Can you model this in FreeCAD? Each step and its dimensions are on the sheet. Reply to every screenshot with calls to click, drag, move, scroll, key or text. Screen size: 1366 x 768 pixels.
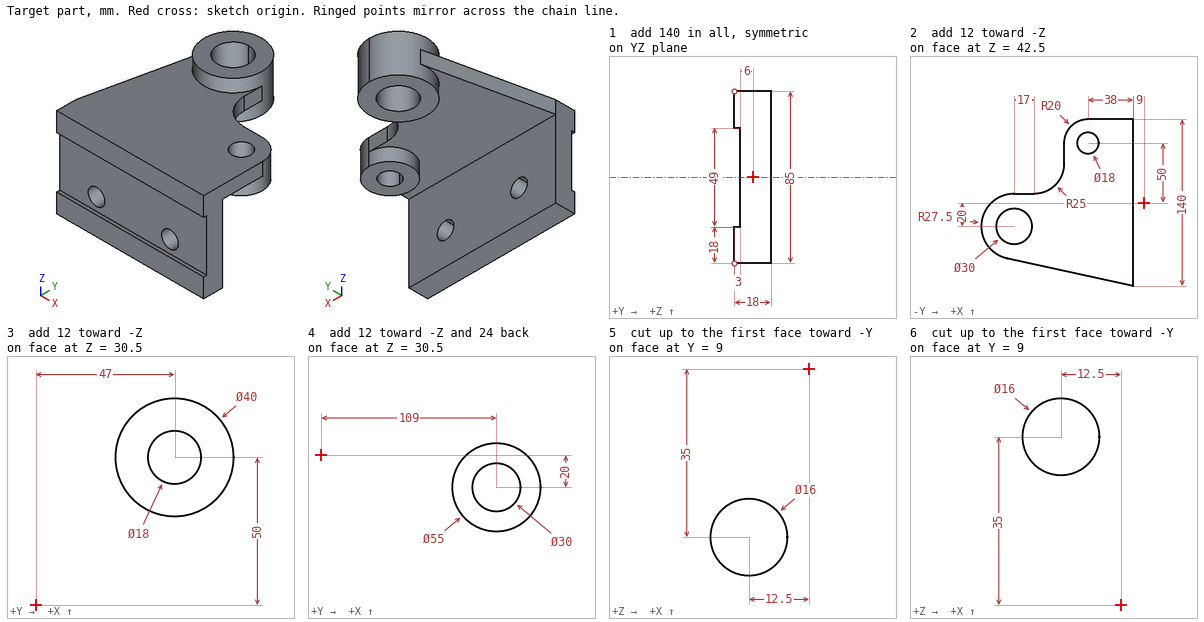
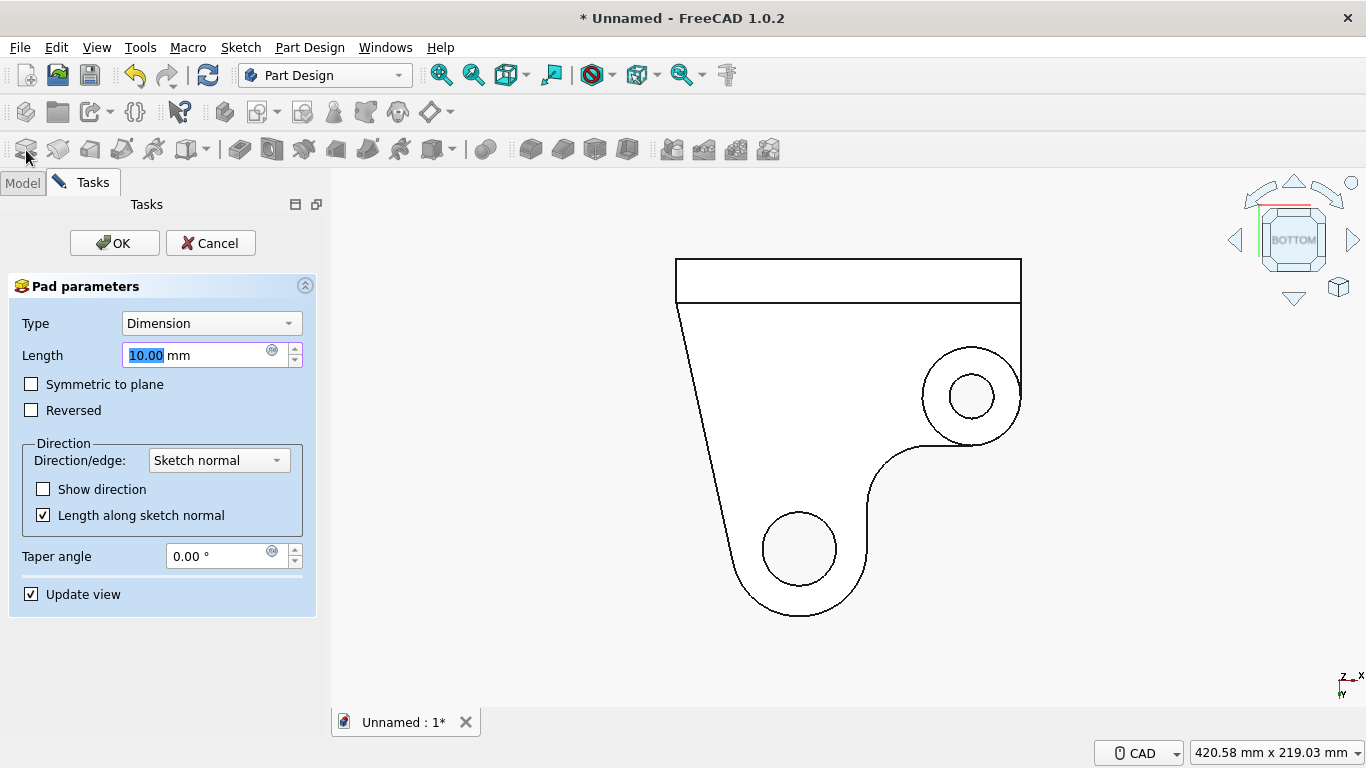
text(12)
key(Tab)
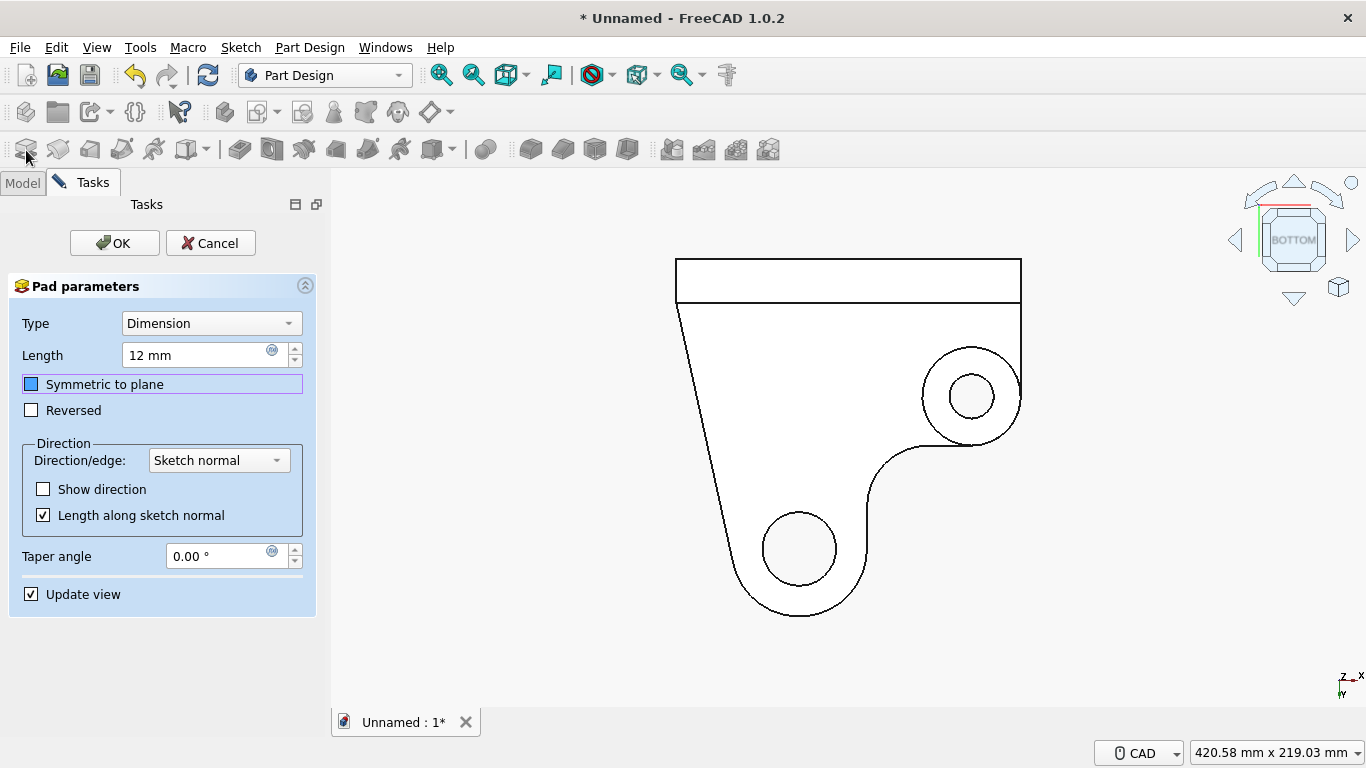
click(115, 243)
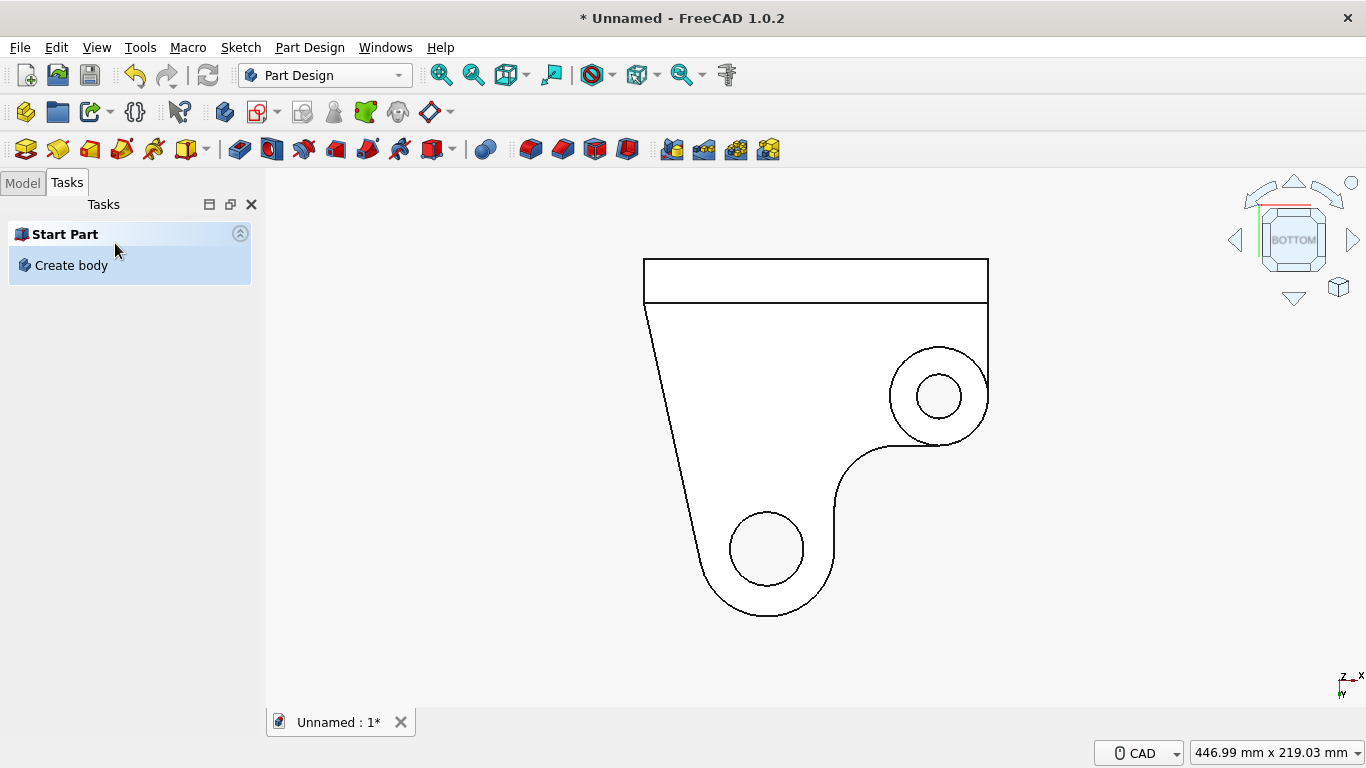
click(767, 414)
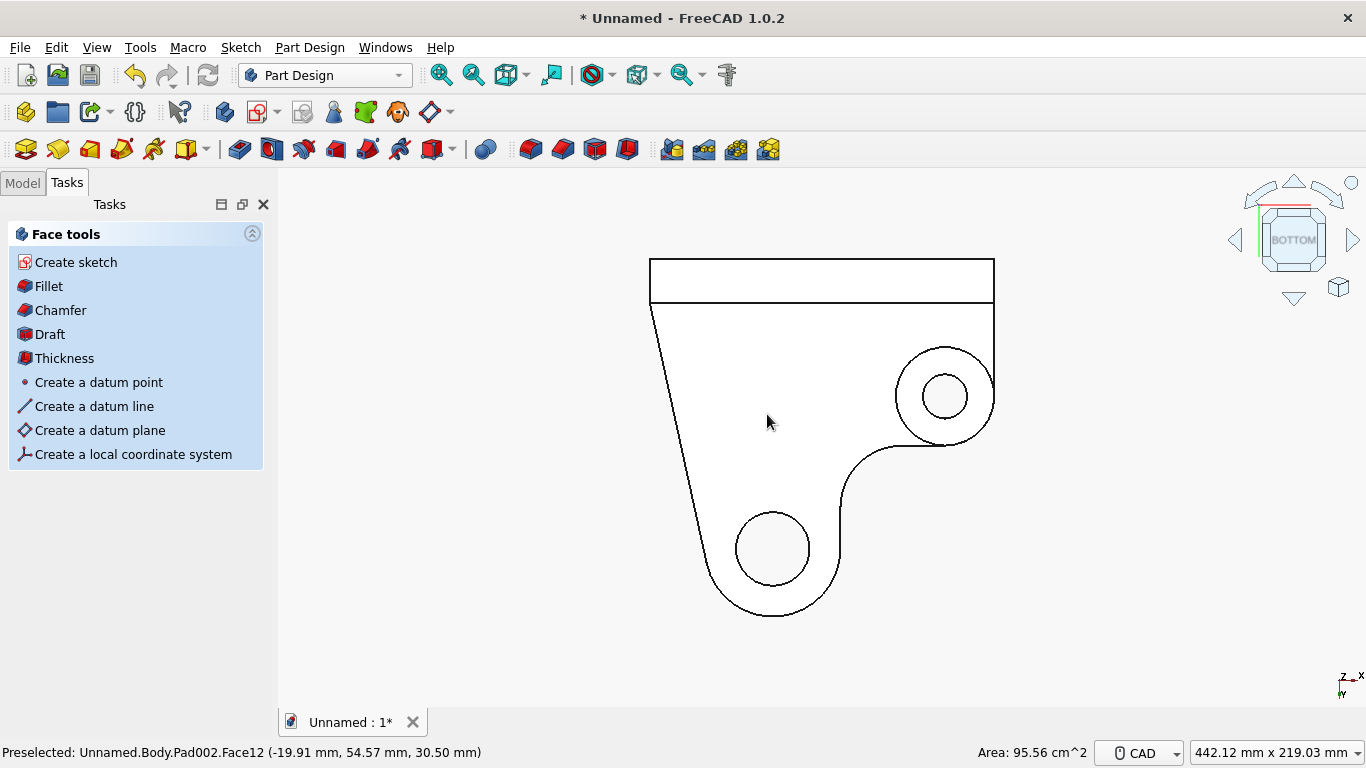
click(258, 112)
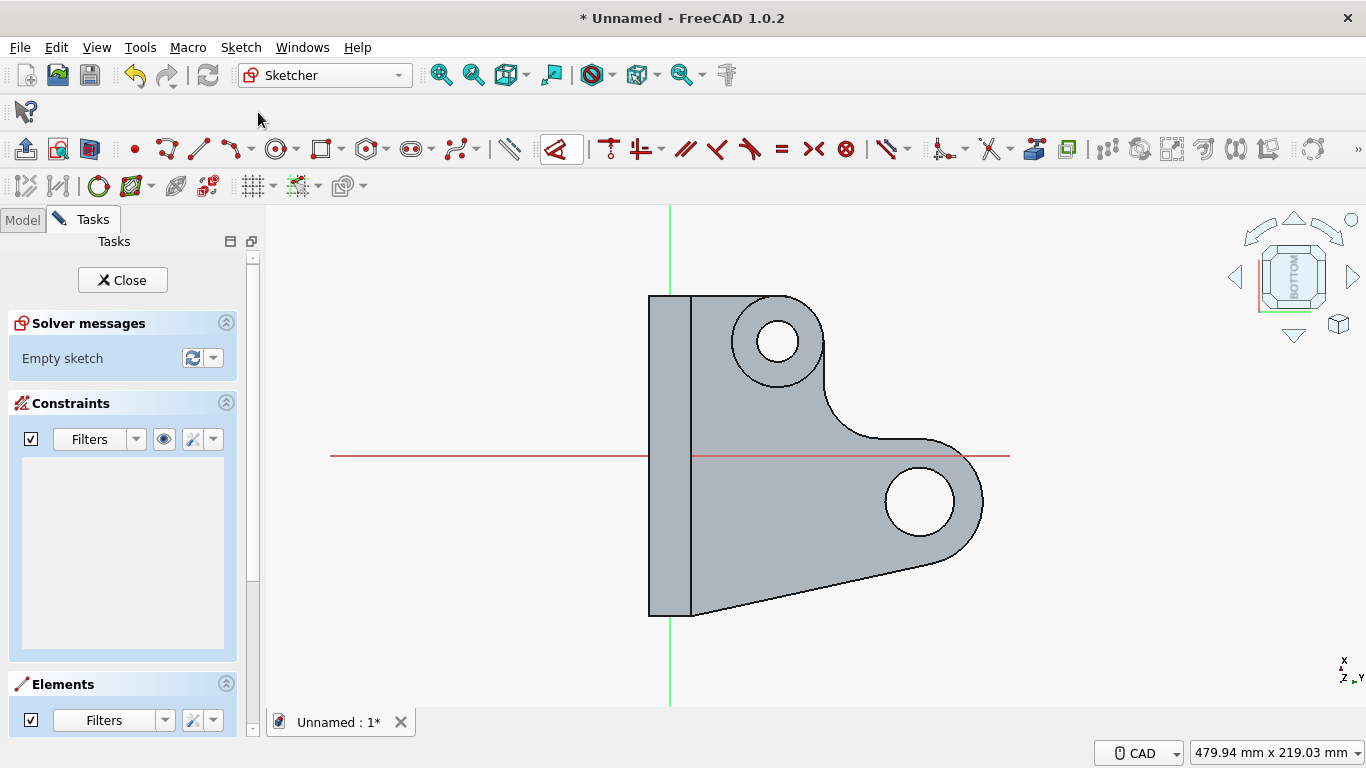
scroll(891, 539, up, 4)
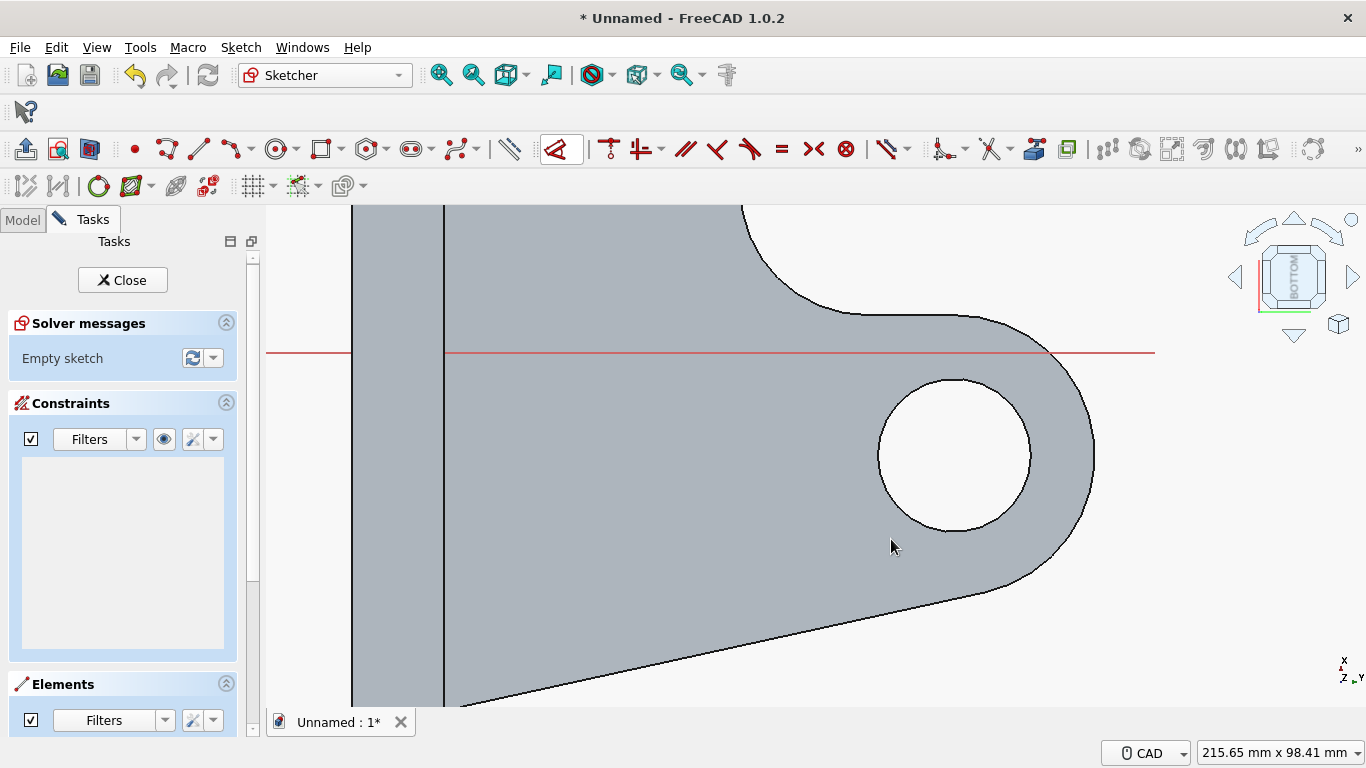
key(g)
key(c)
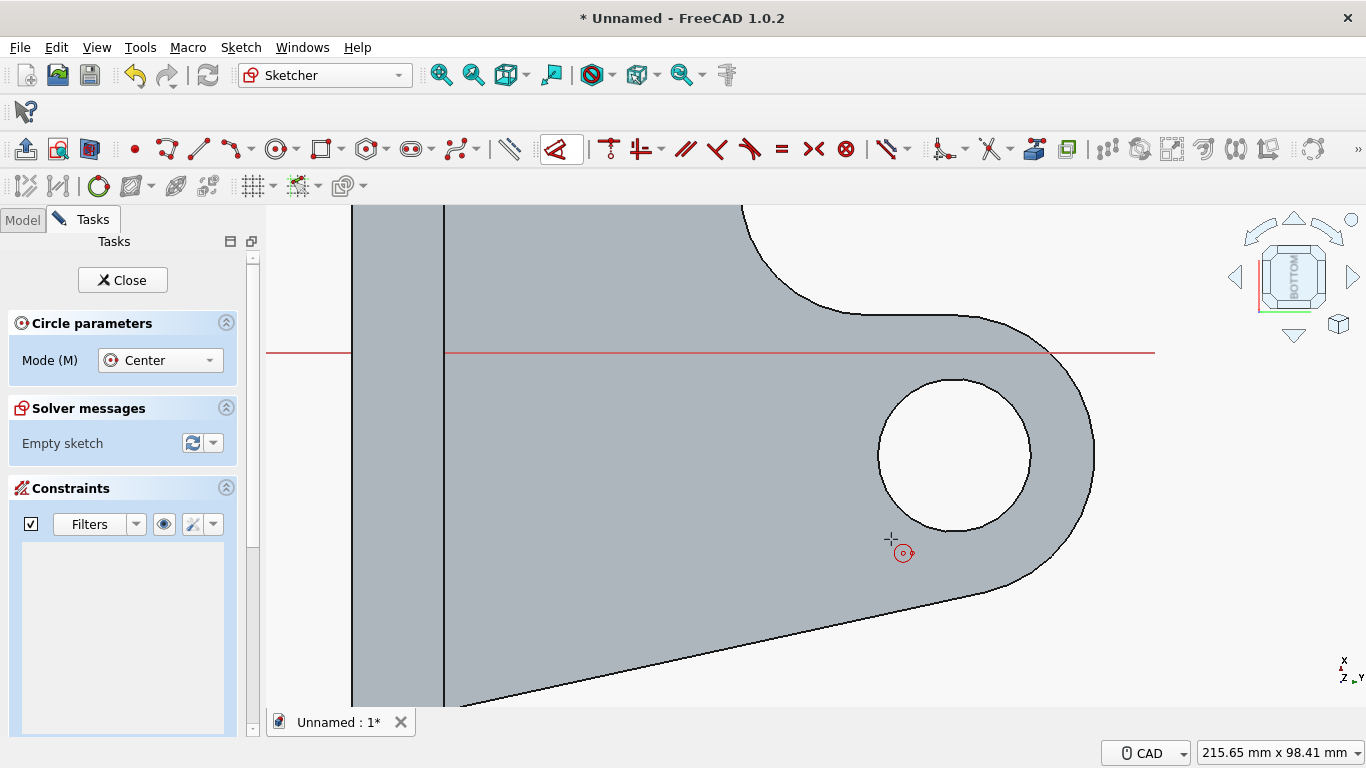
click(954, 455)
move(1054, 555)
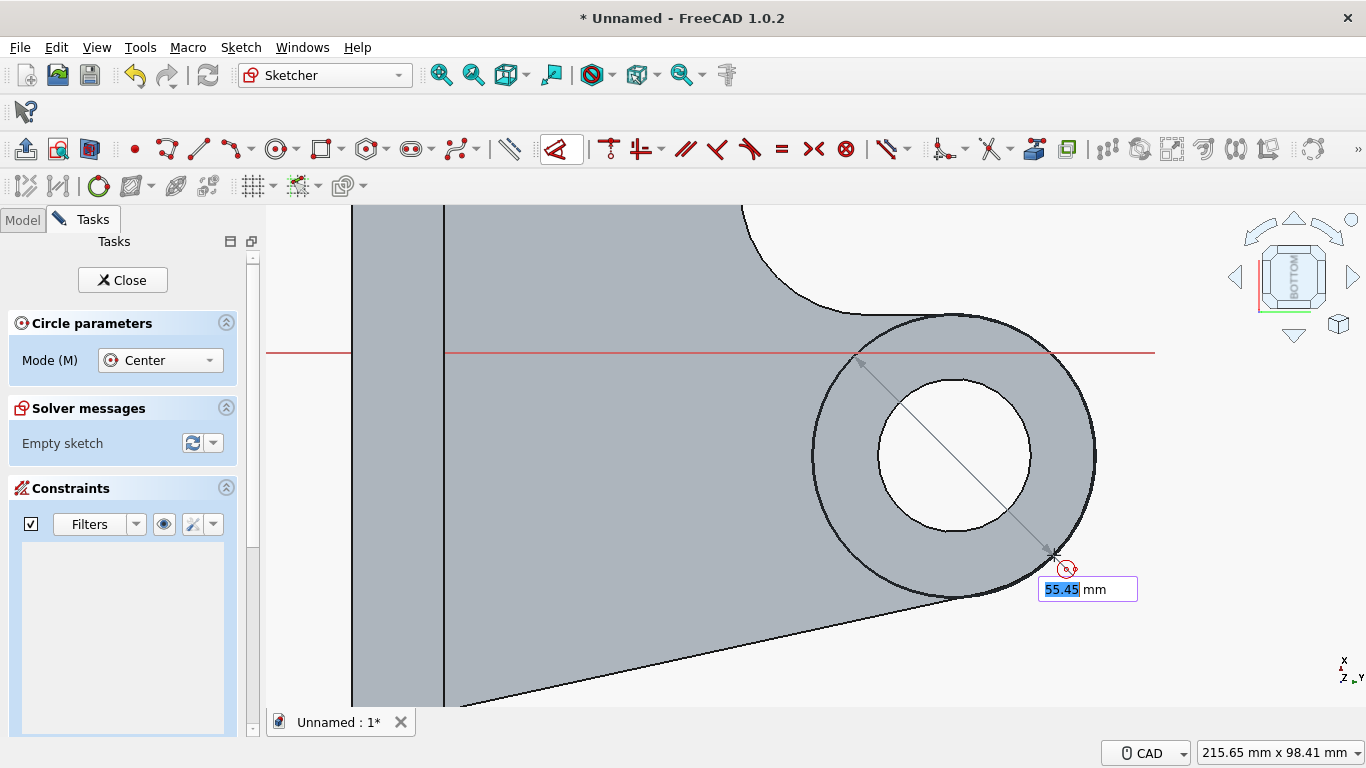
text(55)
key(Return)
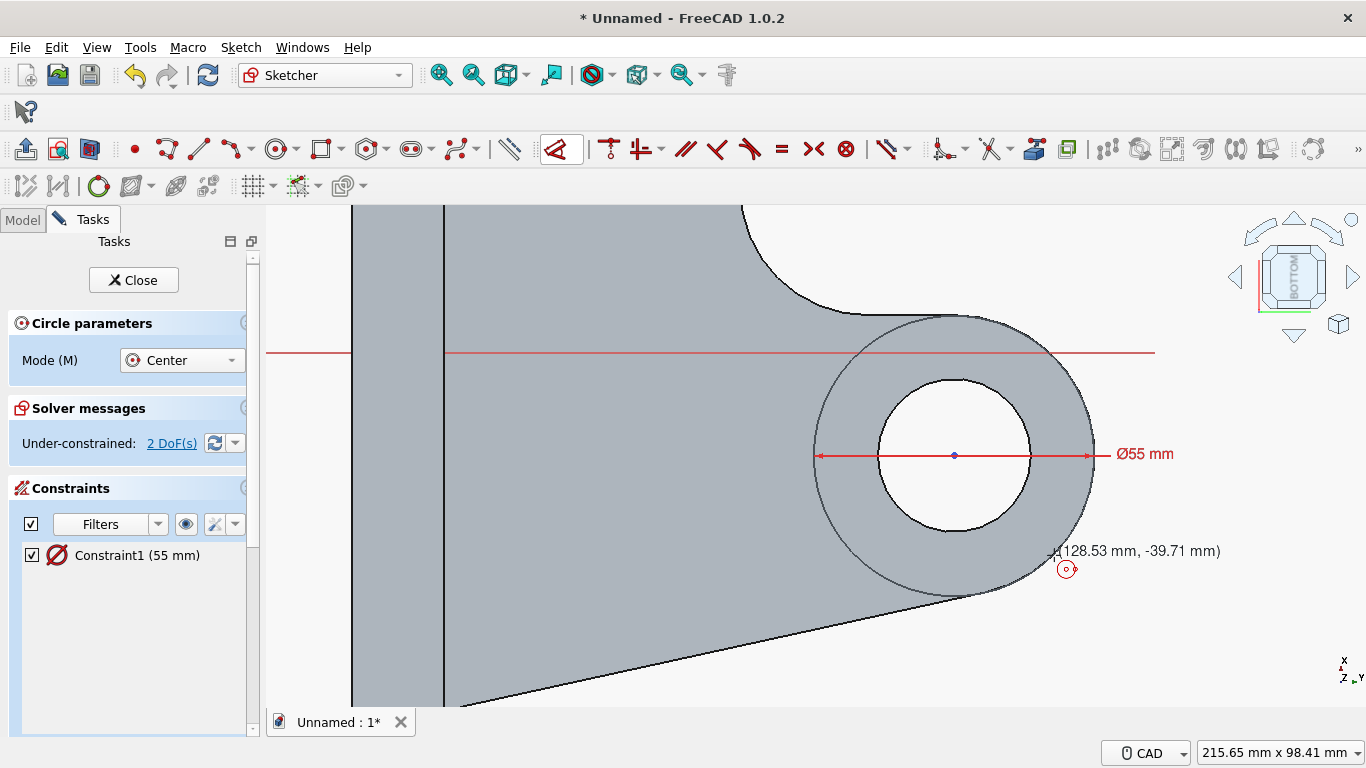
click(954, 456)
move(1009, 401)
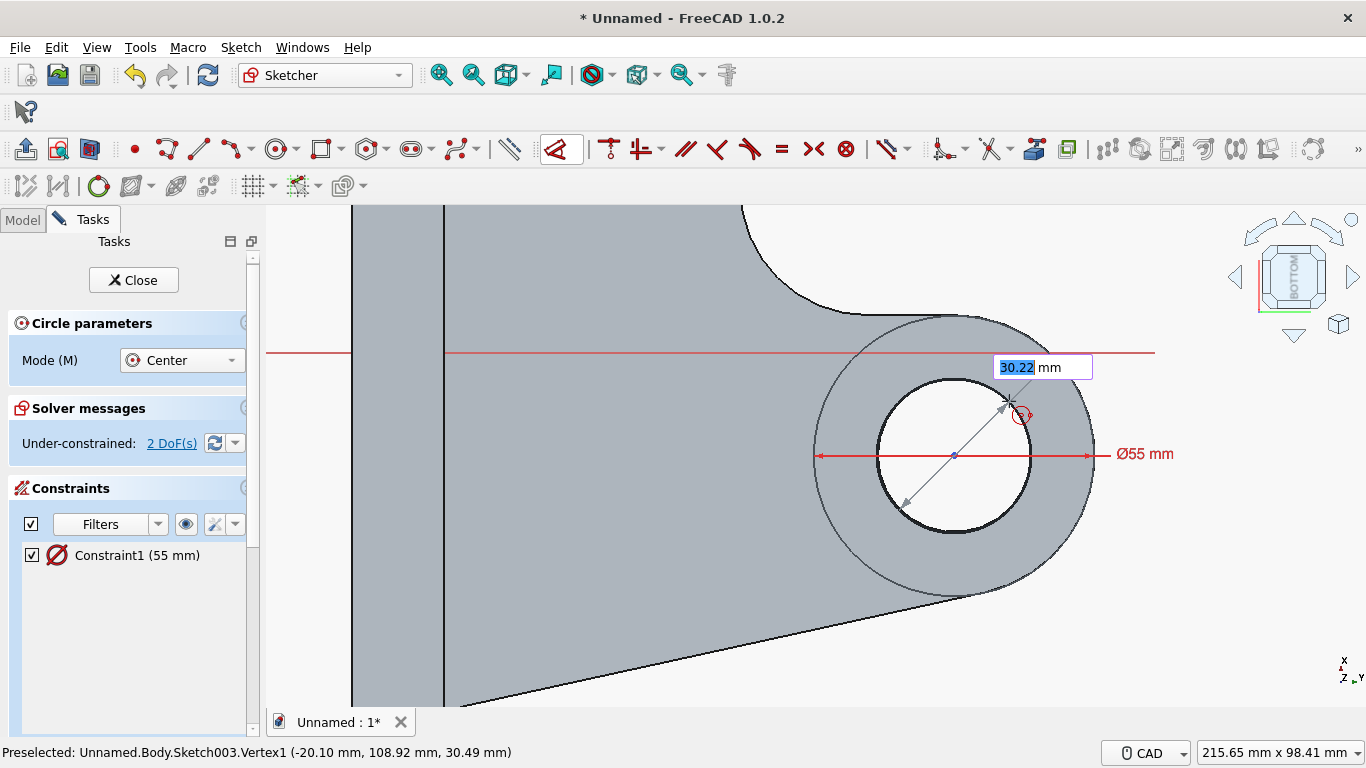
text(30)
key(Return)
key(Escape)